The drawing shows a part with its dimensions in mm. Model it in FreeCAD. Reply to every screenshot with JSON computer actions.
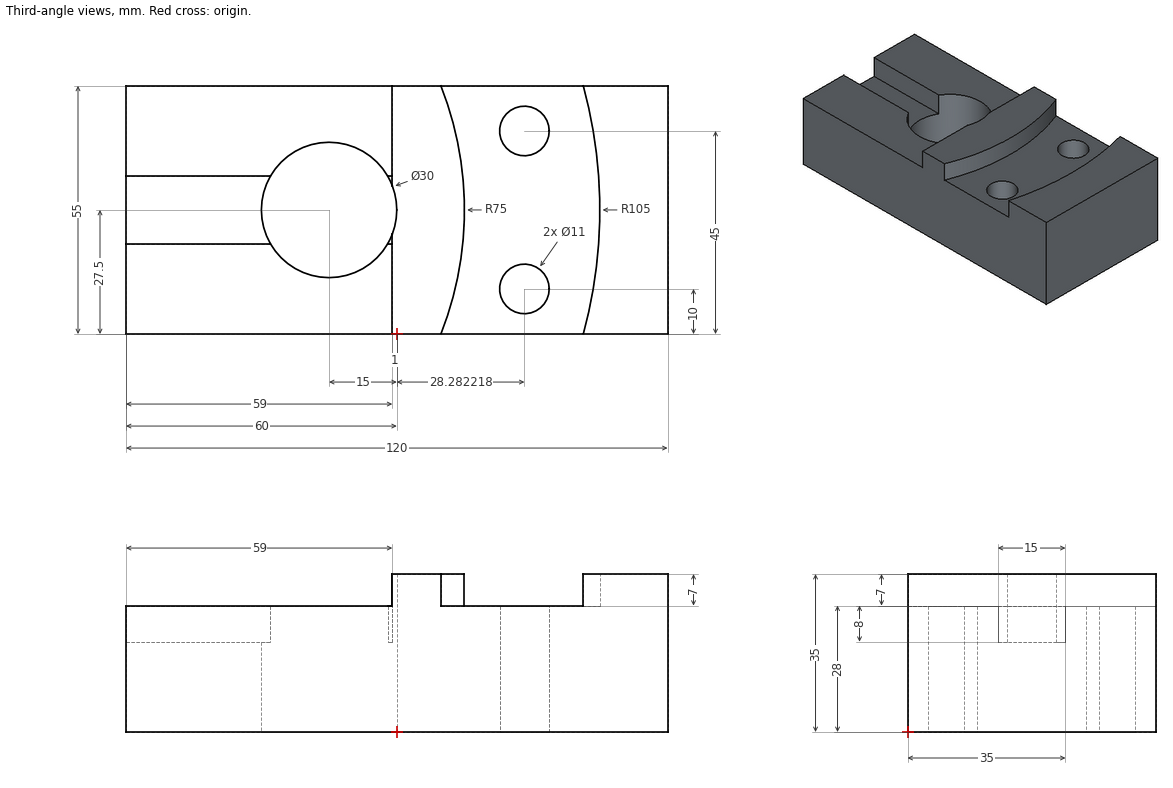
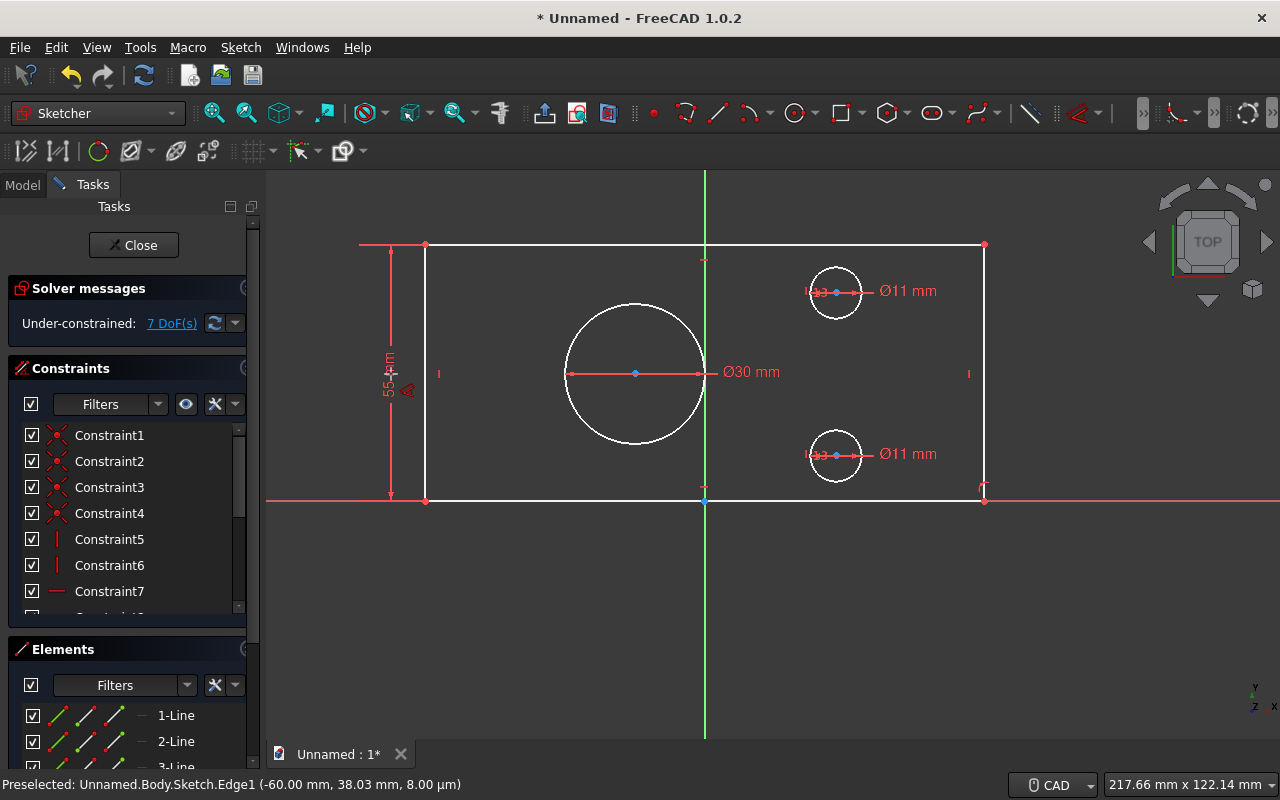
{"action": "left_click", "coordinate": [836, 456]}
{"action": "left_click", "coordinate": [870, 479]}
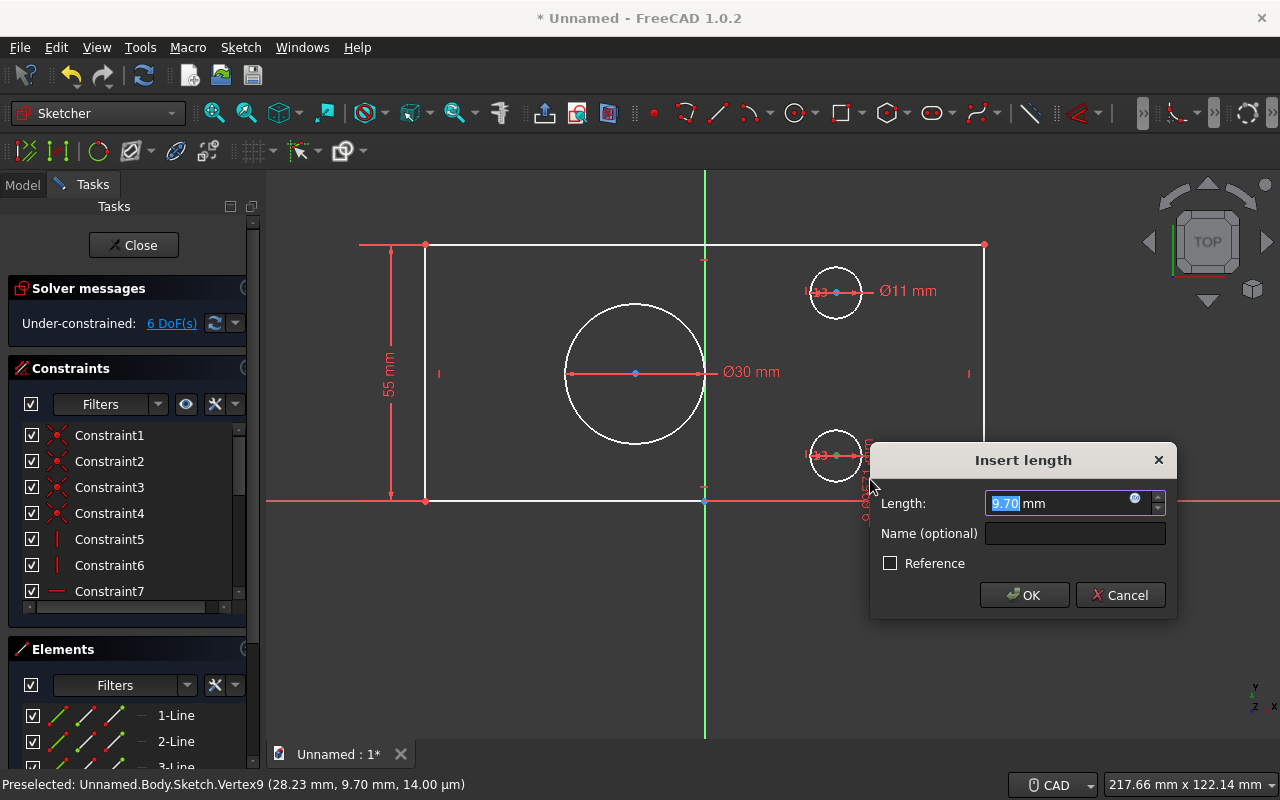
{"action": "type", "text": "10"}
{"action": "key", "text": "Return"}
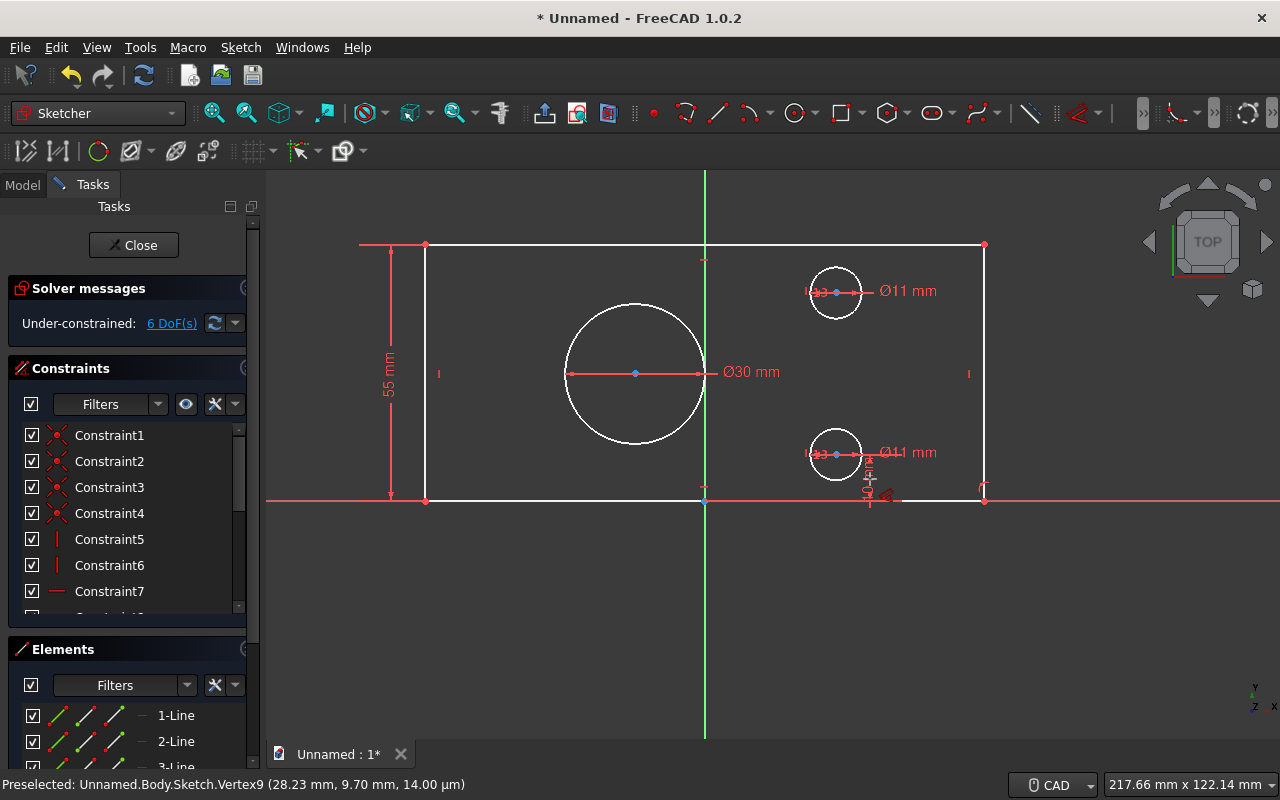
{"action": "left_click", "coordinate": [635, 374]}
{"action": "left_click", "coordinate": [670, 535]}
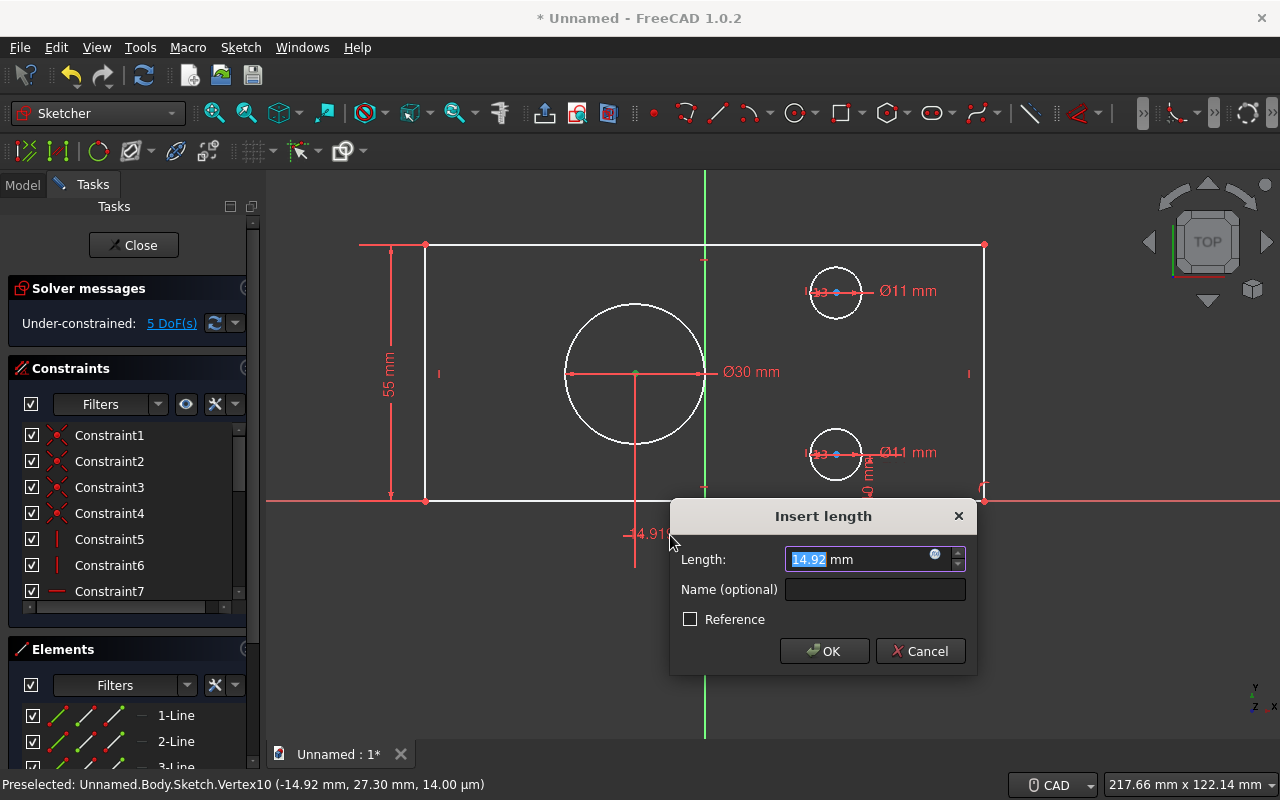
{"action": "type", "text": "15"}
{"action": "key", "text": "Return"}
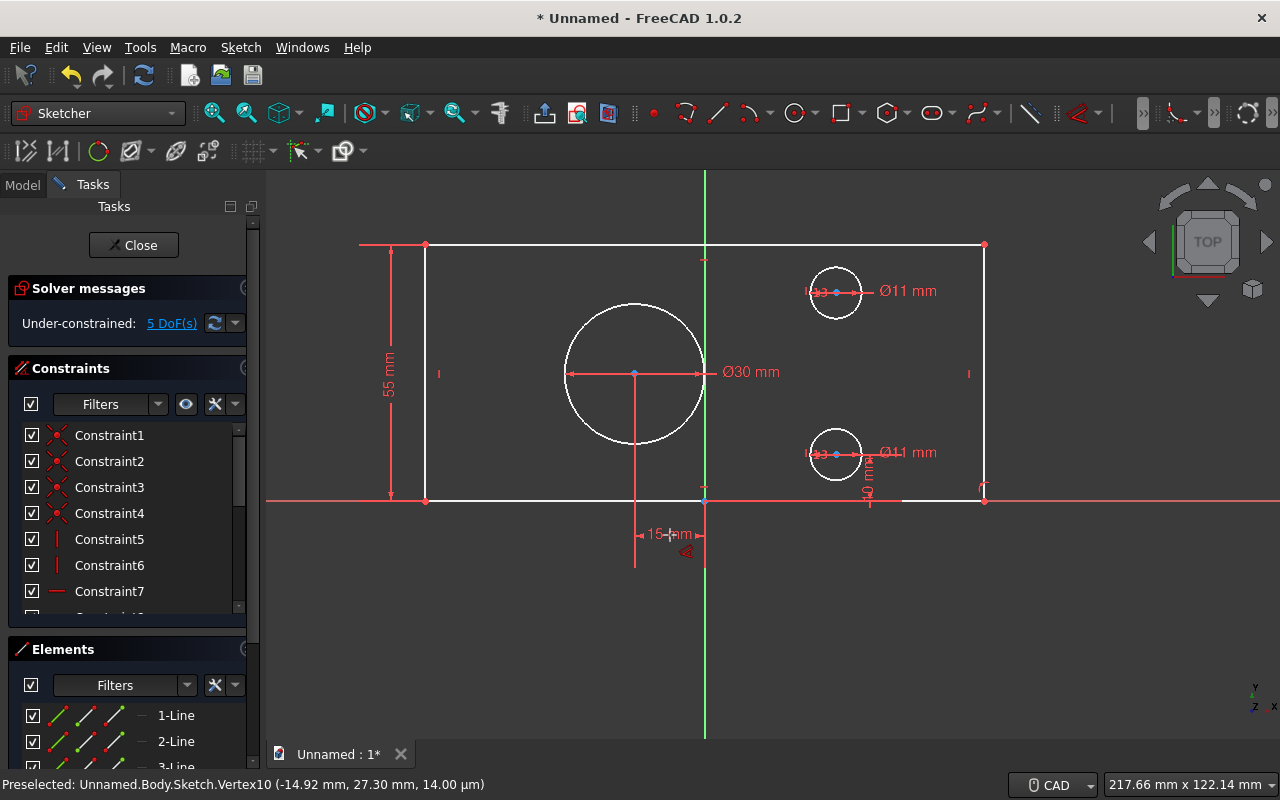
{"action": "left_click", "coordinate": [836, 293]}
{"action": "left_click", "coordinate": [870, 397]}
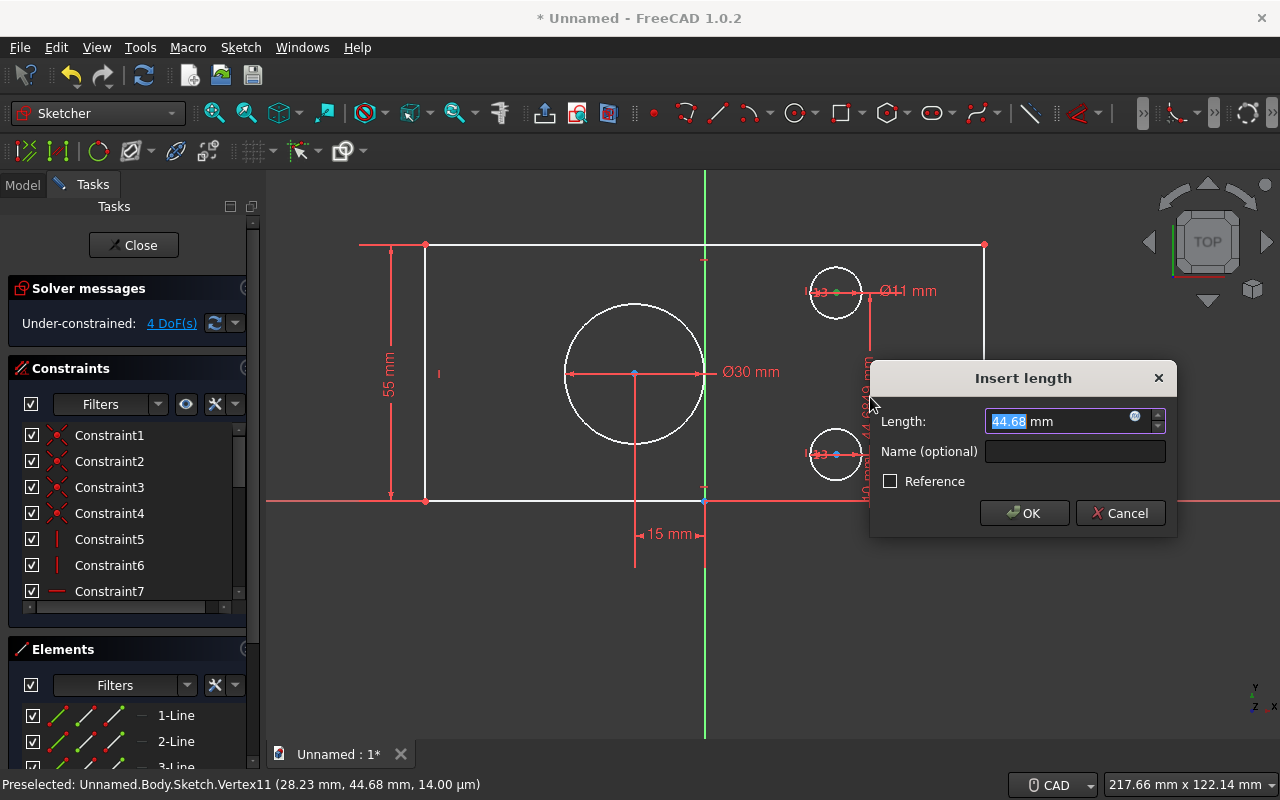
{"action": "type", "text": "45"}
{"action": "key", "text": "Return"}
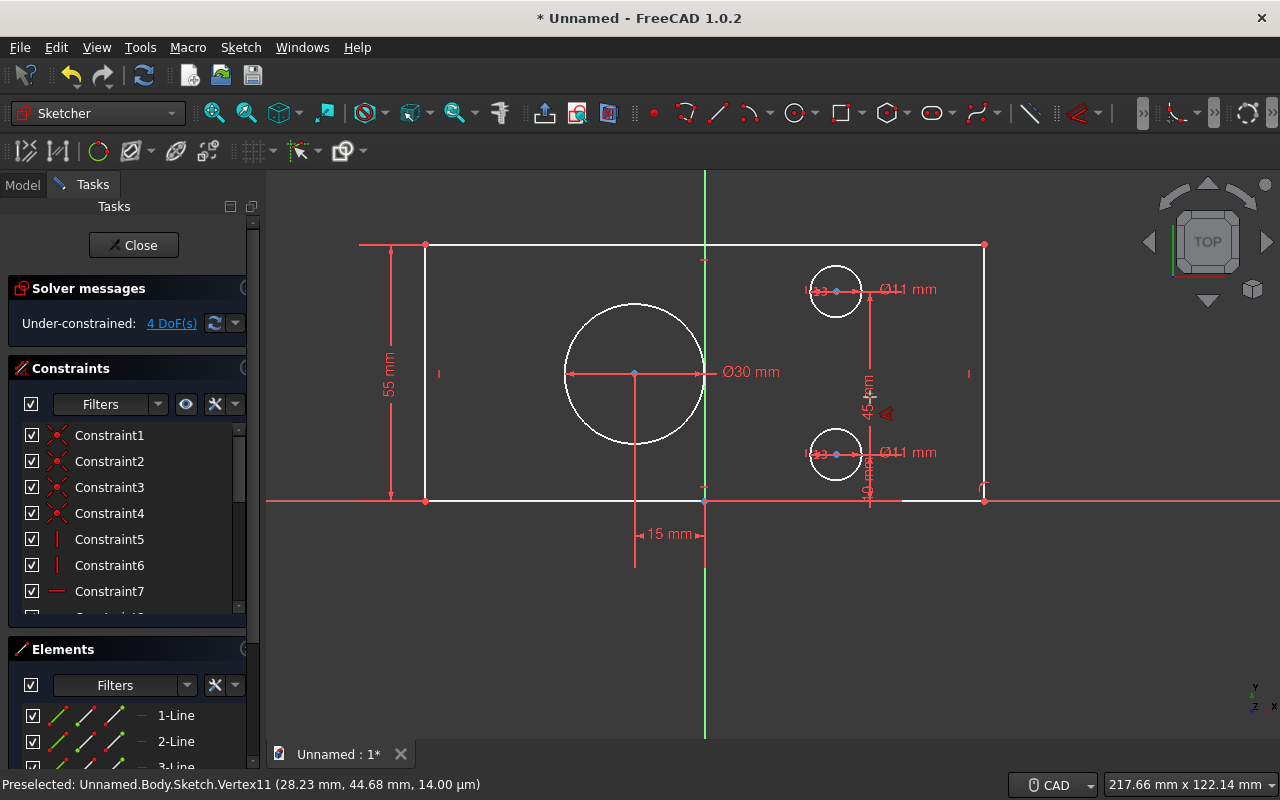
{"action": "left_click", "coordinate": [593, 501]}
{"action": "left_click", "coordinate": [576, 535]}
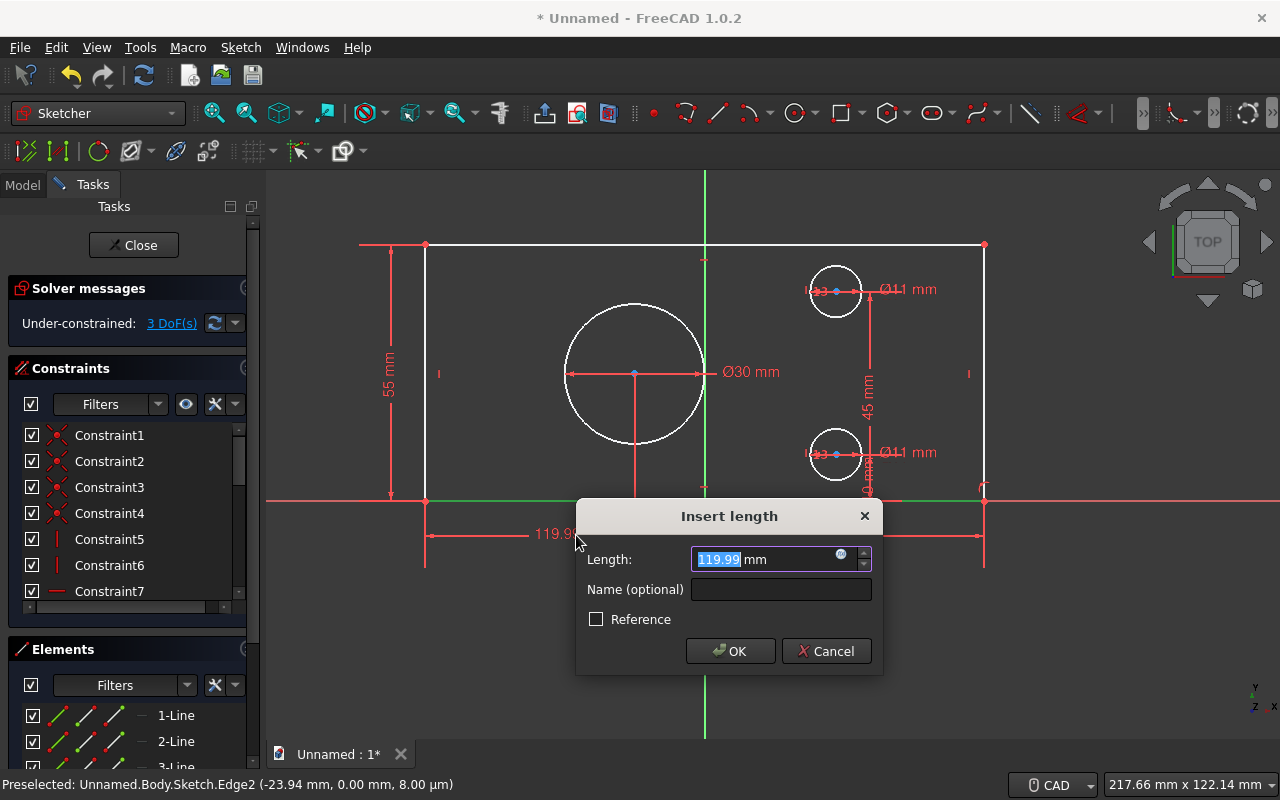
{"action": "type", "text": "120"}
{"action": "key", "text": "Return"}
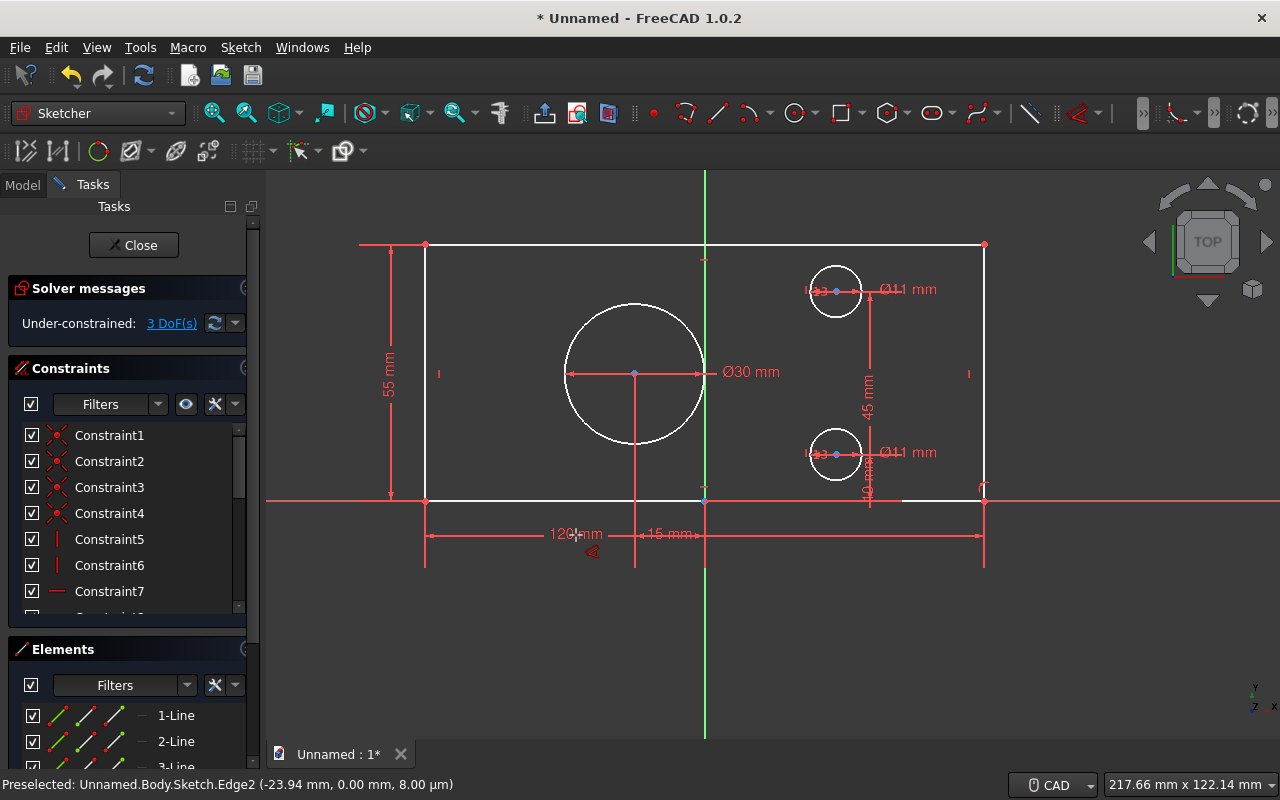
{"action": "left_click", "coordinate": [425, 245]}
{"action": "left_click", "coordinate": [500, 535]}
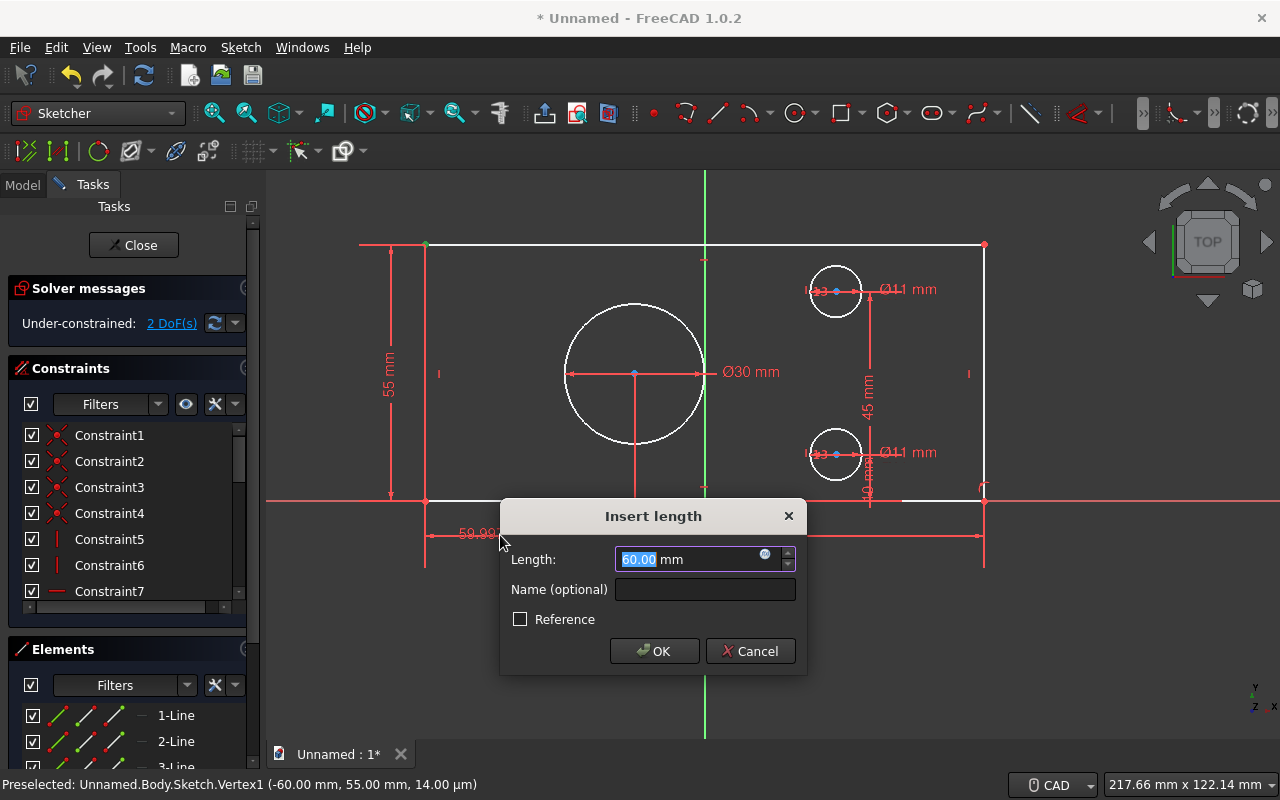
{"action": "type", "text": "60"}
{"action": "key", "text": "Return"}